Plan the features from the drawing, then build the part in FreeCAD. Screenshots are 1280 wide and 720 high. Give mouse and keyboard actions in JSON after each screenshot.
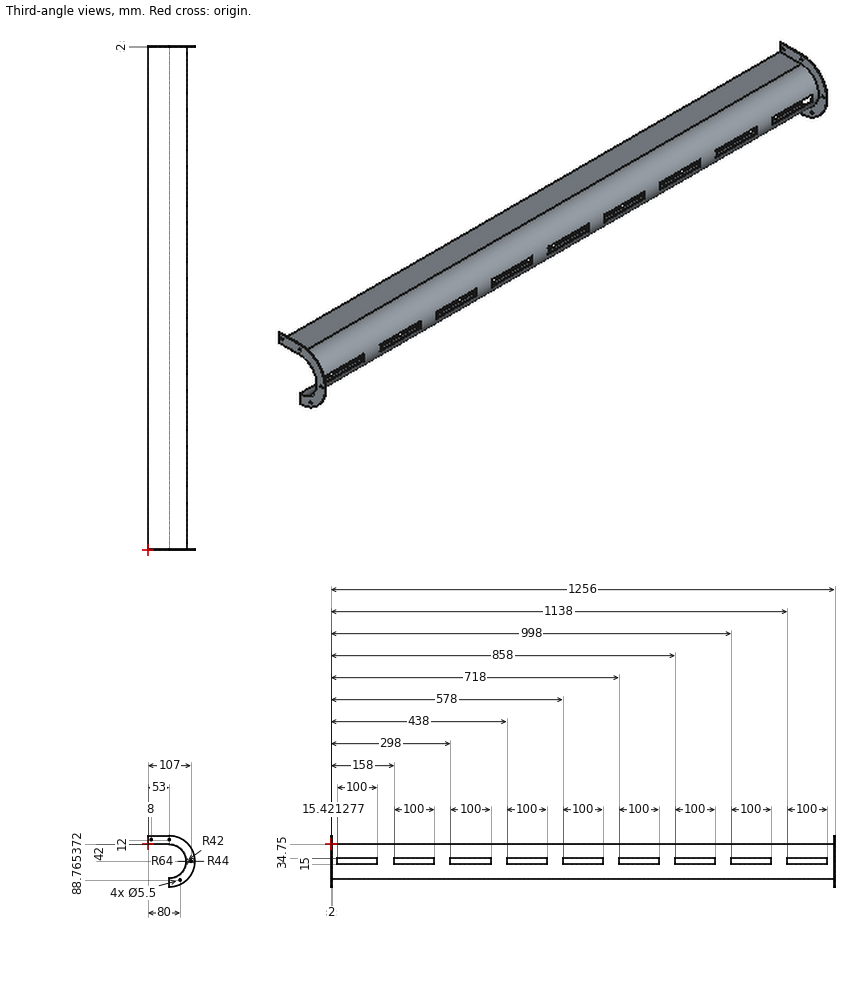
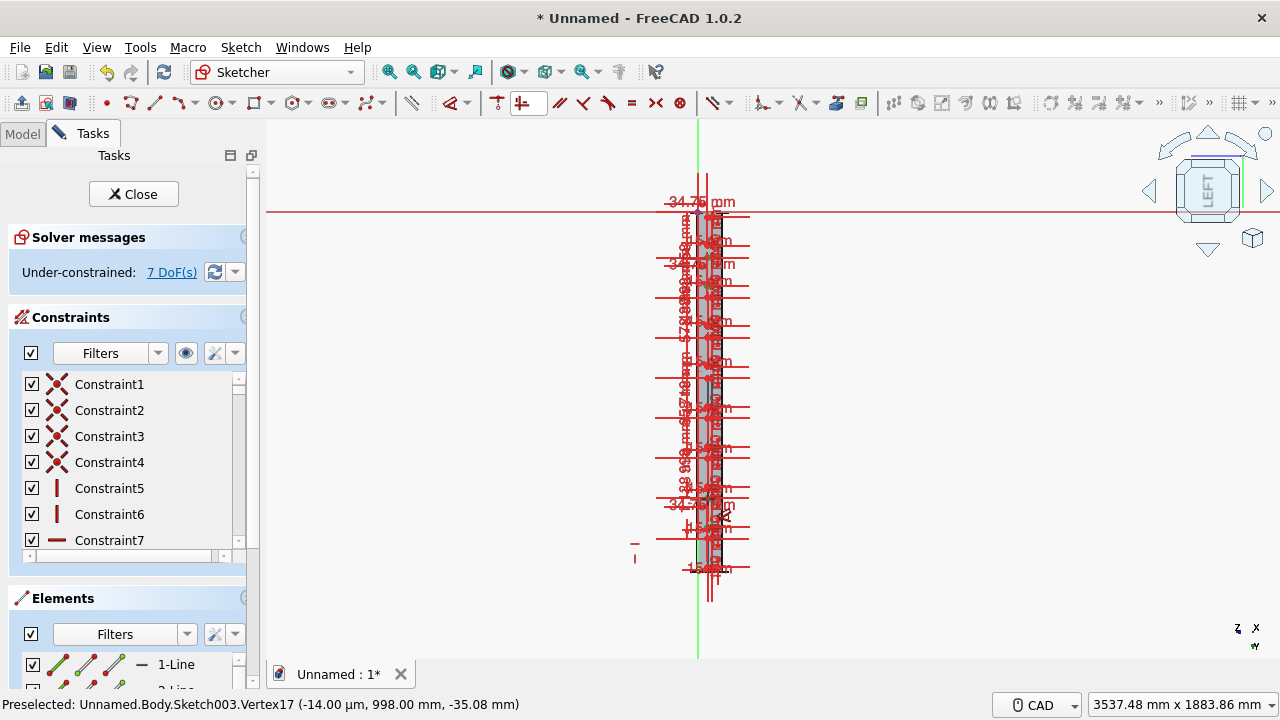
{"action": "scroll", "coordinate": [708, 298], "scroll_direction": "up", "scroll_amount": 7}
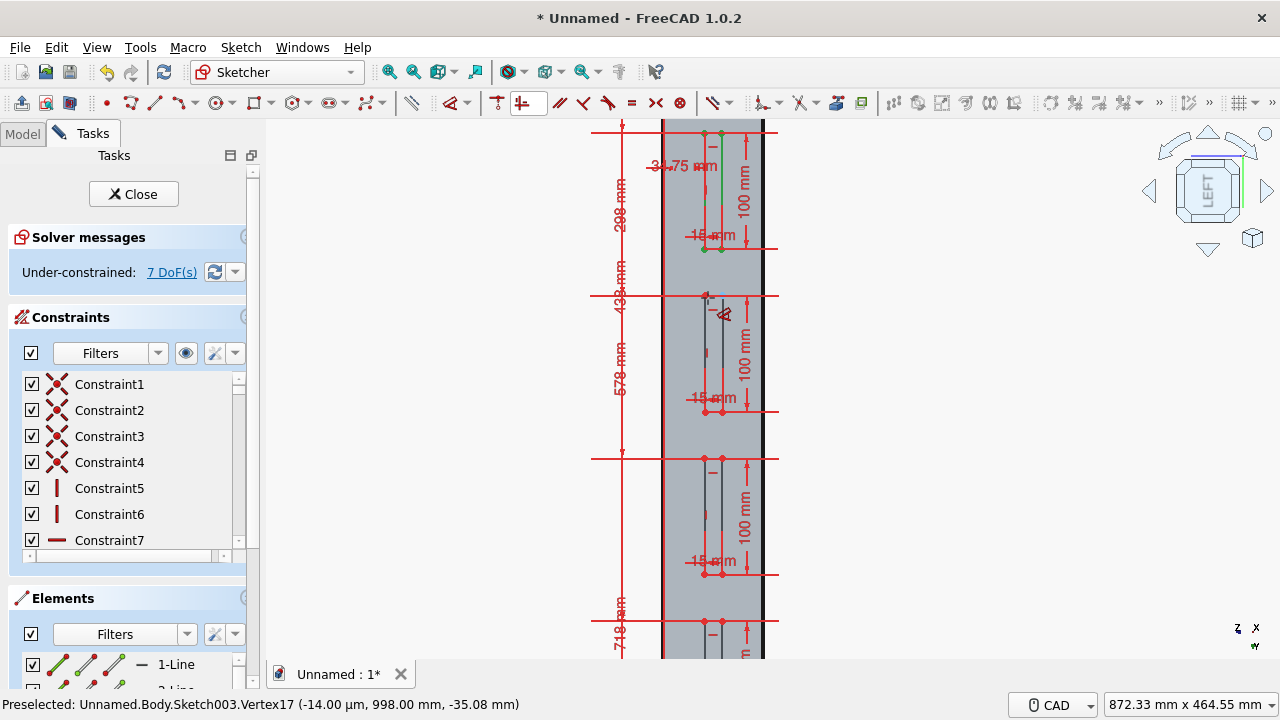
{"action": "left_click", "coordinate": [705, 296]}
{"action": "left_click", "coordinate": [685, 330]}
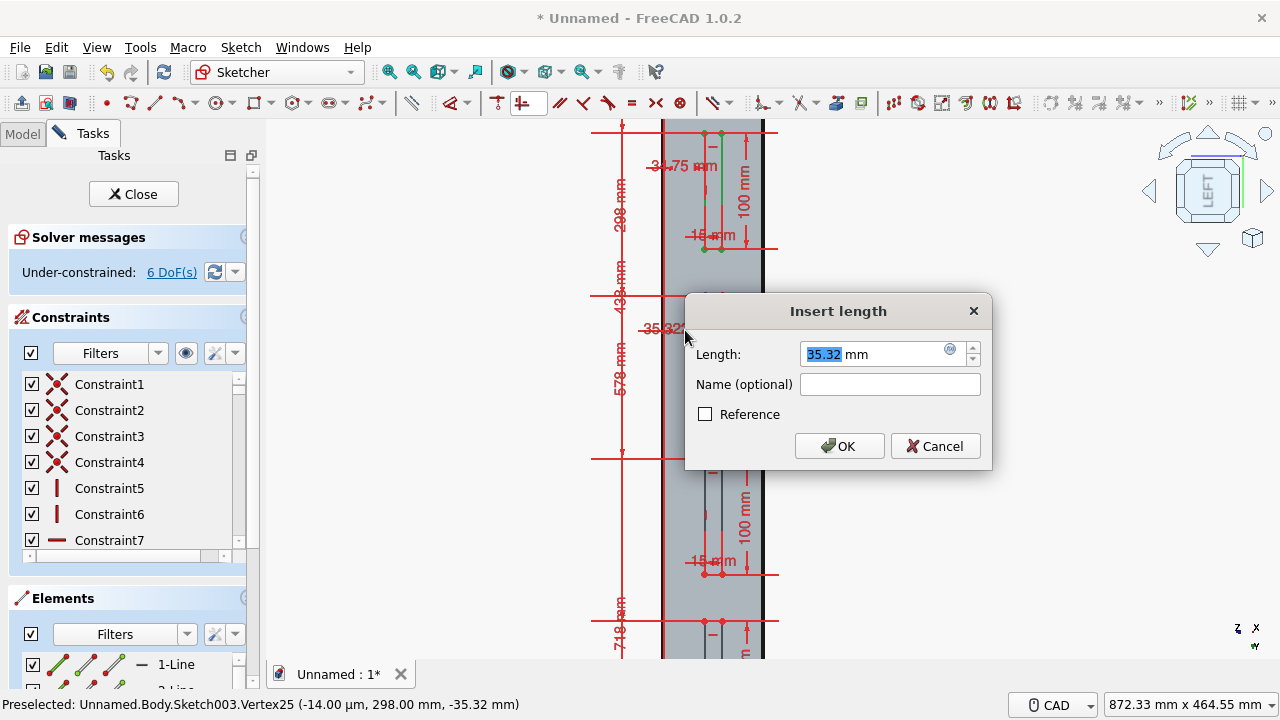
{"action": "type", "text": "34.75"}
{"action": "key", "text": "Return"}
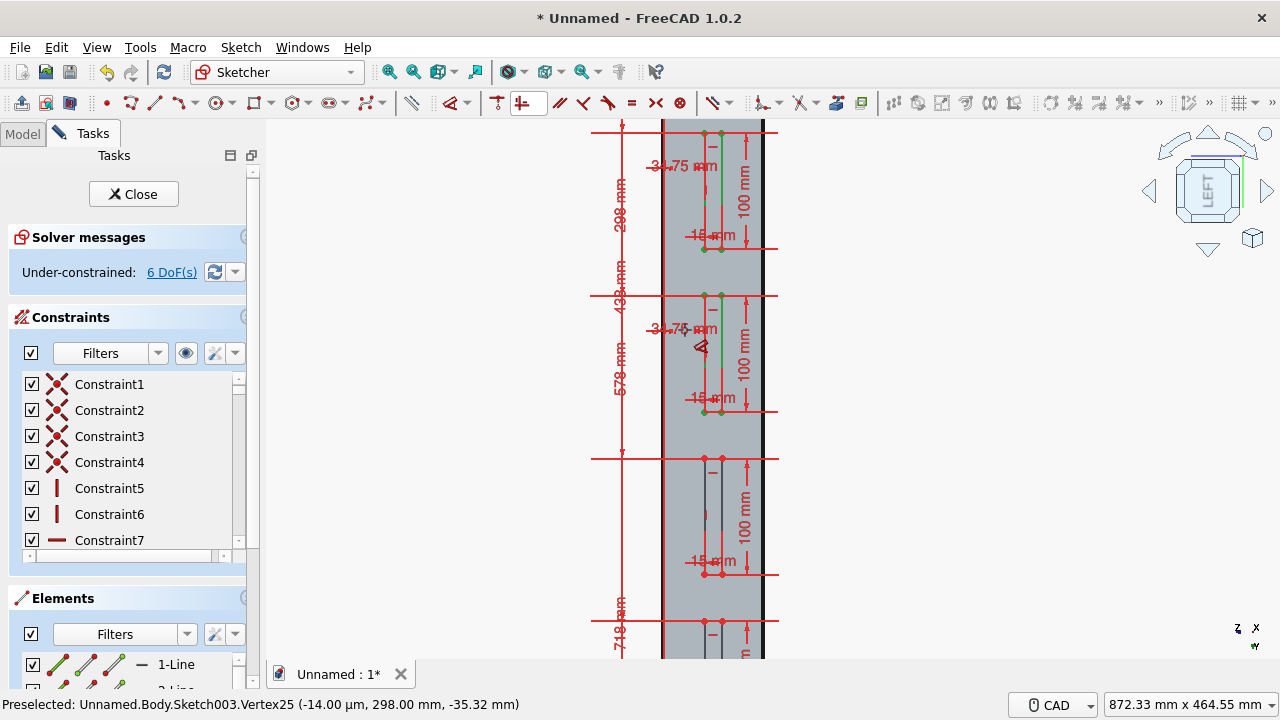
{"action": "left_click", "coordinate": [705, 459]}
{"action": "left_click", "coordinate": [685, 493]}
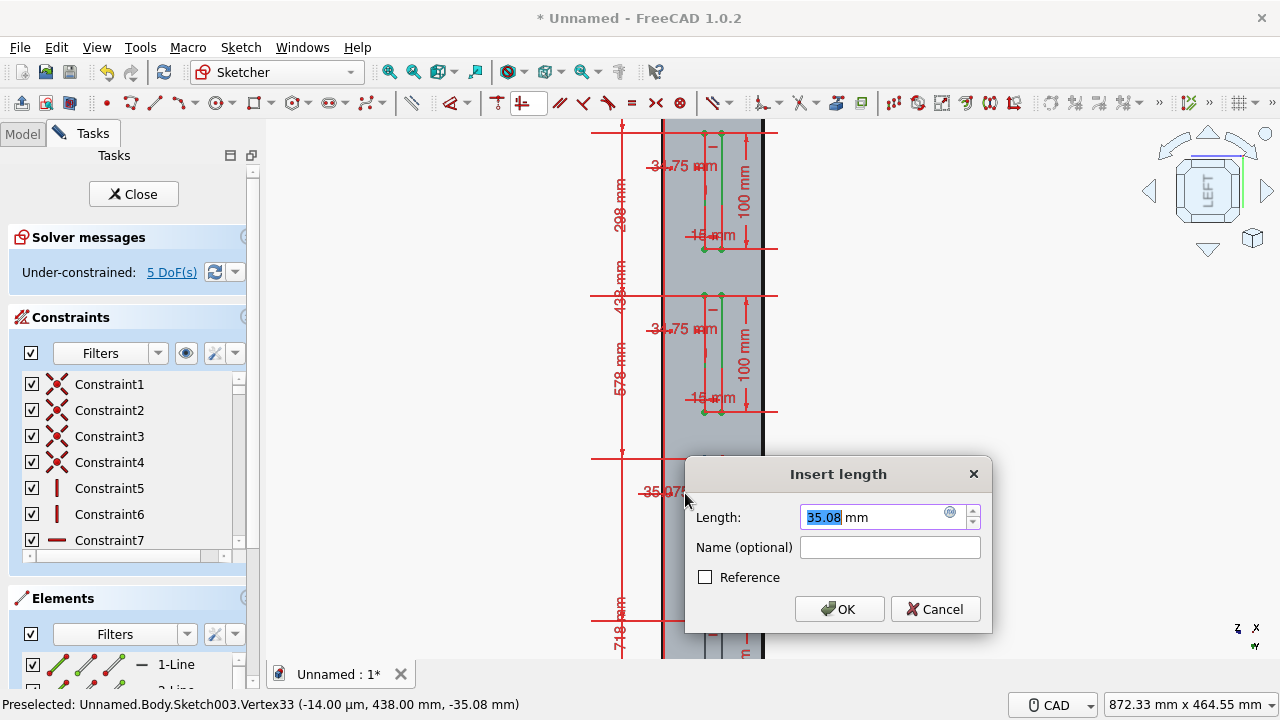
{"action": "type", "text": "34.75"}
{"action": "key", "text": "Return"}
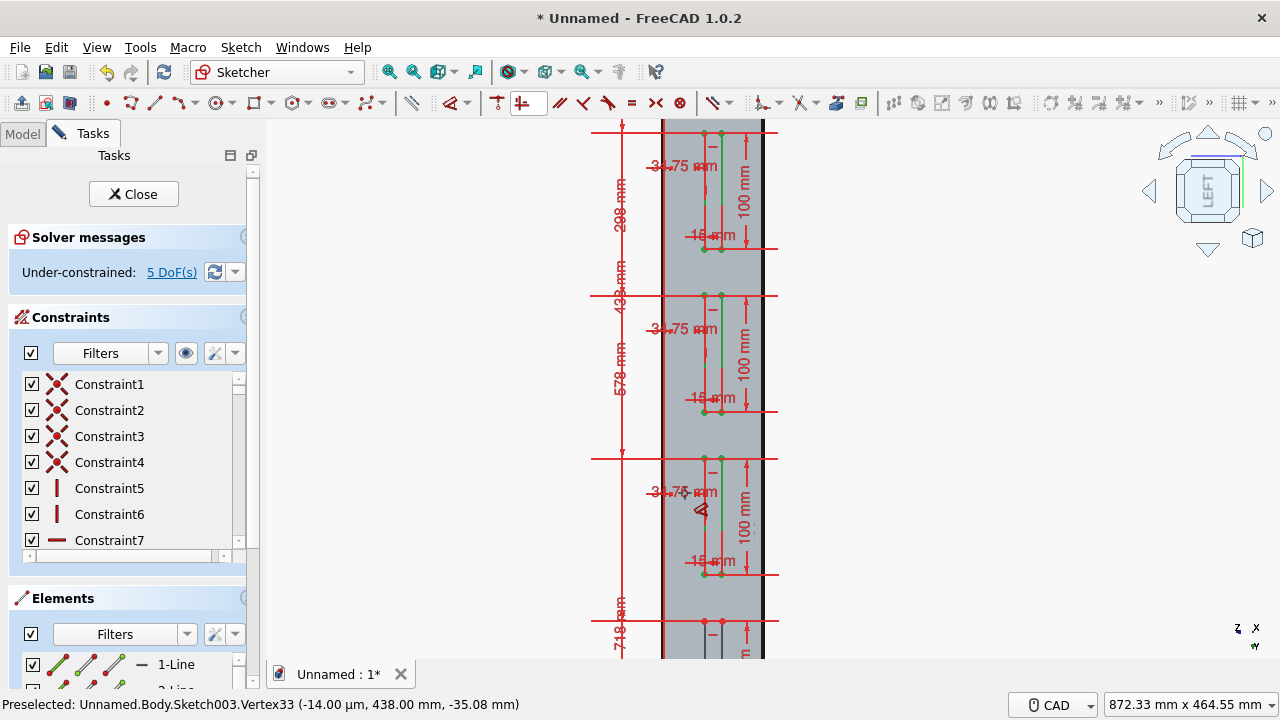
{"action": "left_click", "coordinate": [705, 621]}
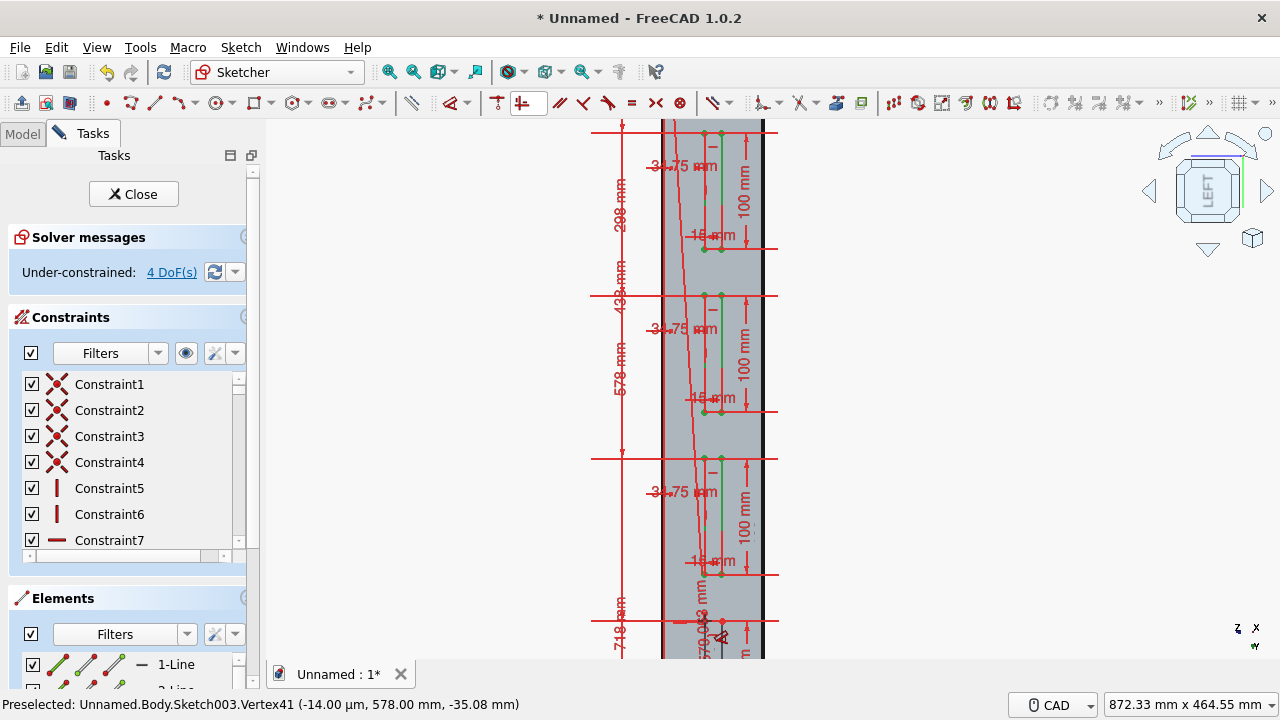
{"action": "key", "text": "Escape"}
{"action": "key", "text": "Escape"}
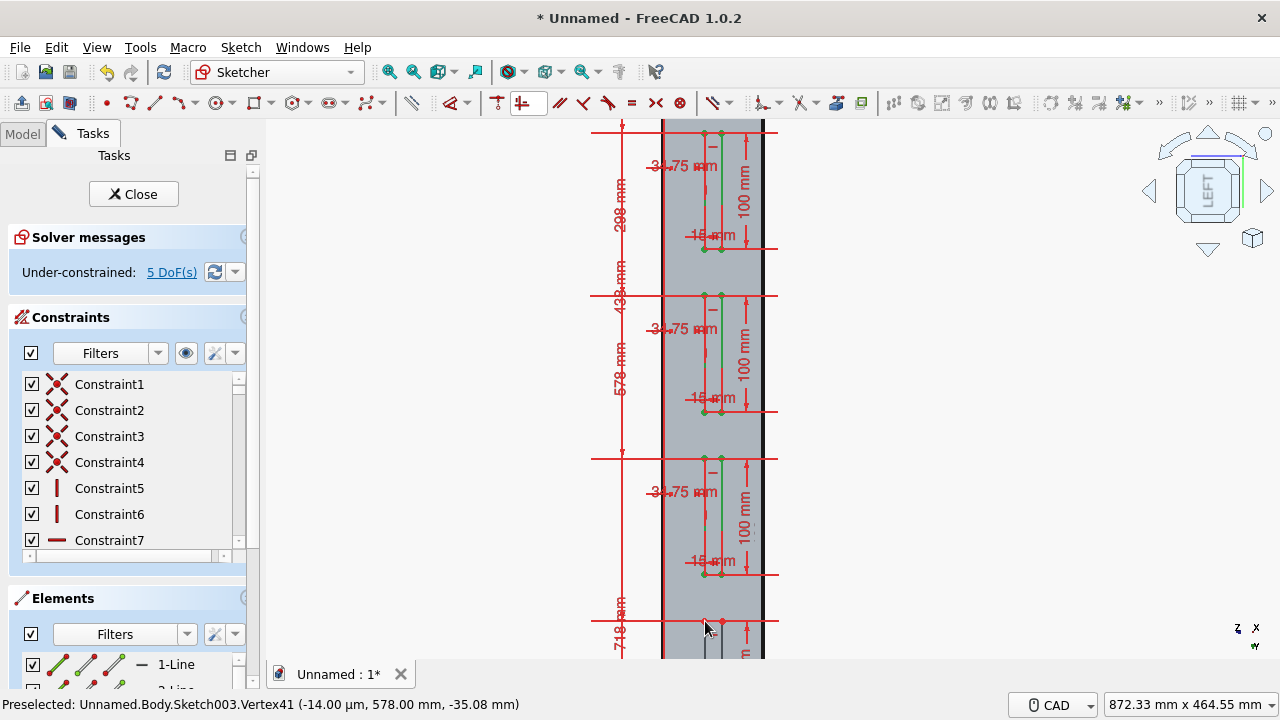
{"action": "left_click", "coordinate": [705, 621]}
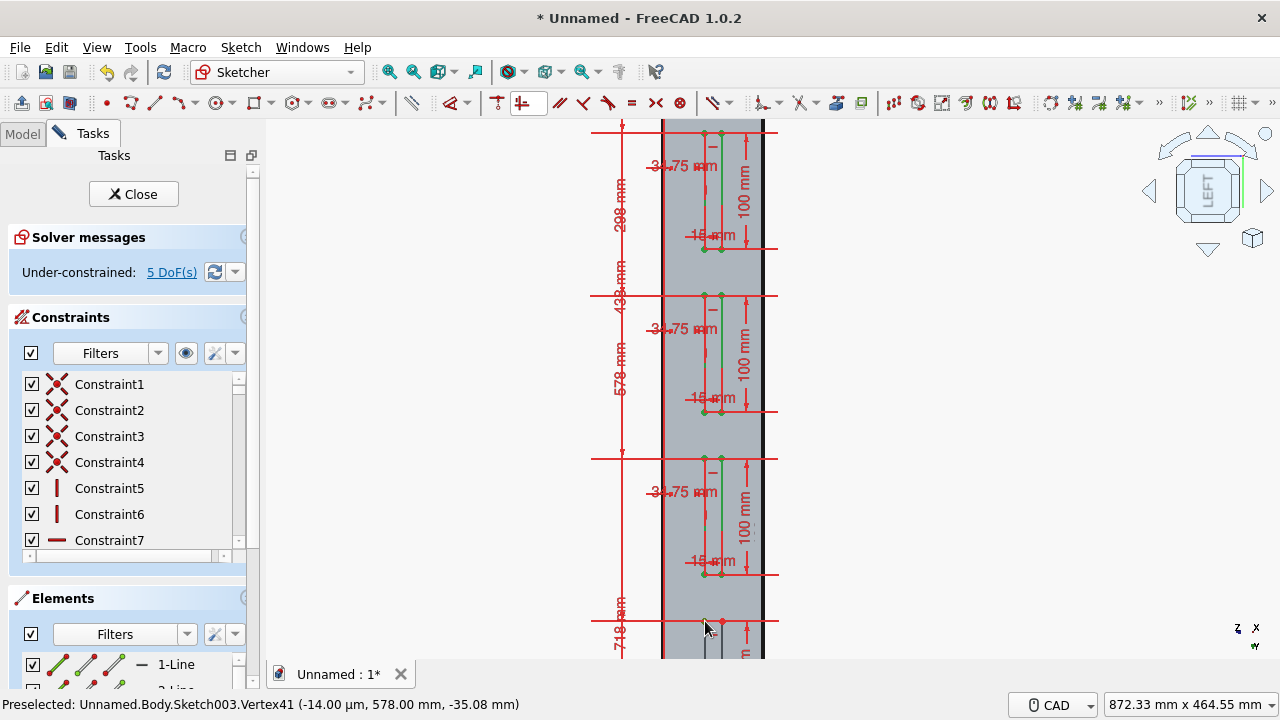
{"action": "key", "text": "l"}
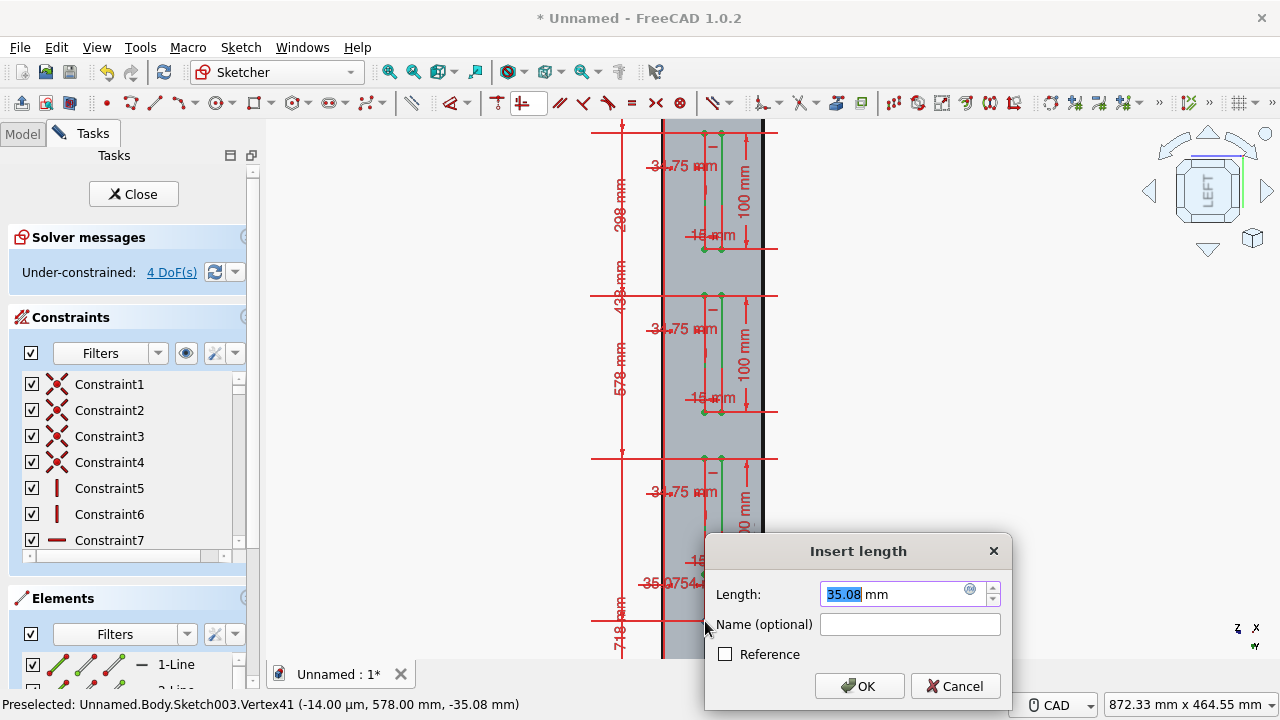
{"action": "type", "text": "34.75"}
{"action": "key", "text": "Return"}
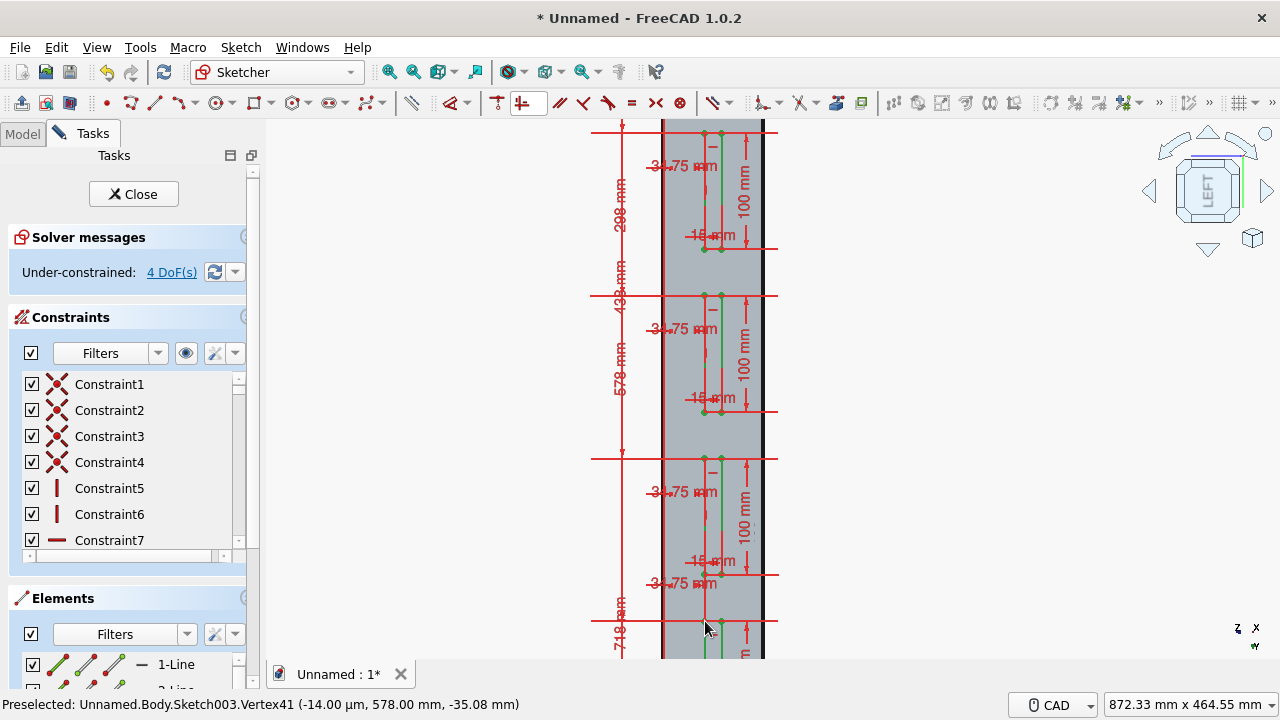
{"action": "scroll", "coordinate": [708, 297], "scroll_direction": "down", "scroll_amount": 7}